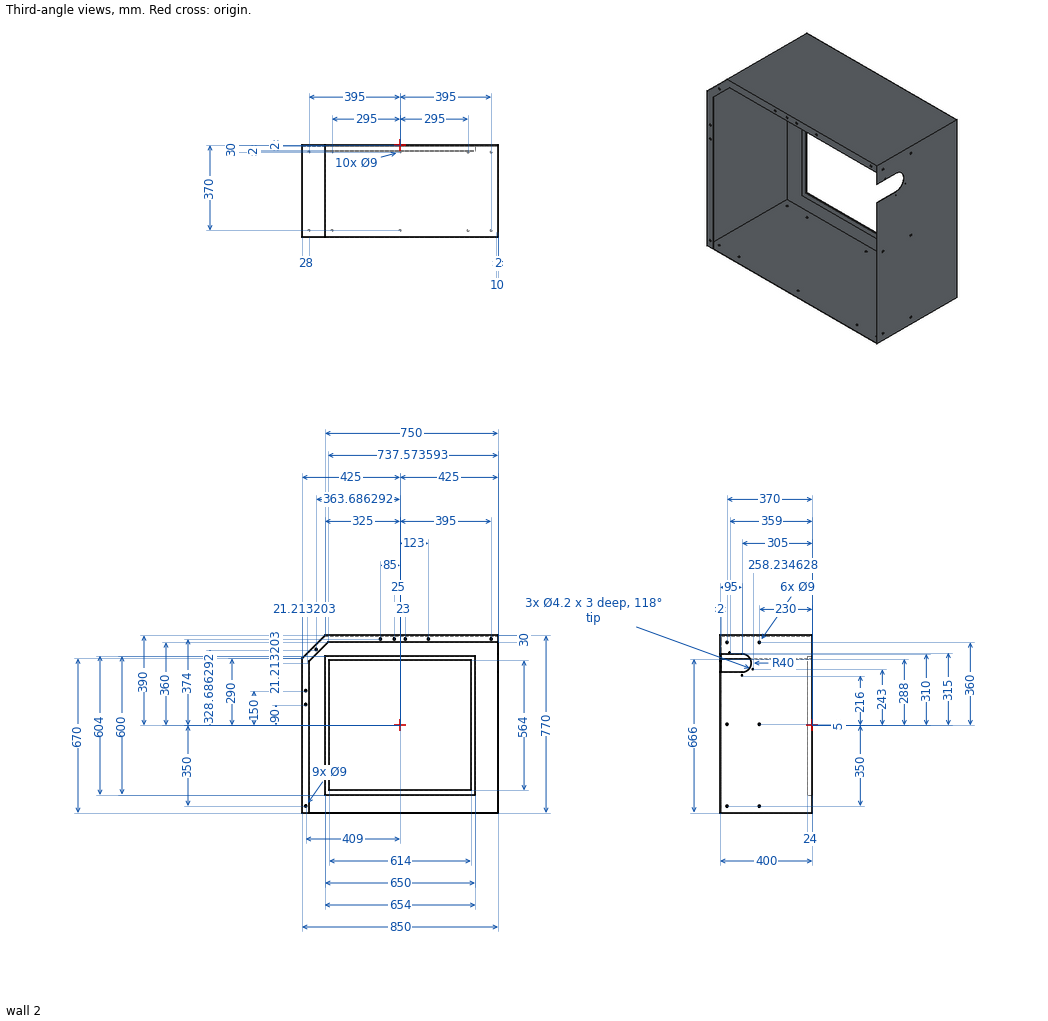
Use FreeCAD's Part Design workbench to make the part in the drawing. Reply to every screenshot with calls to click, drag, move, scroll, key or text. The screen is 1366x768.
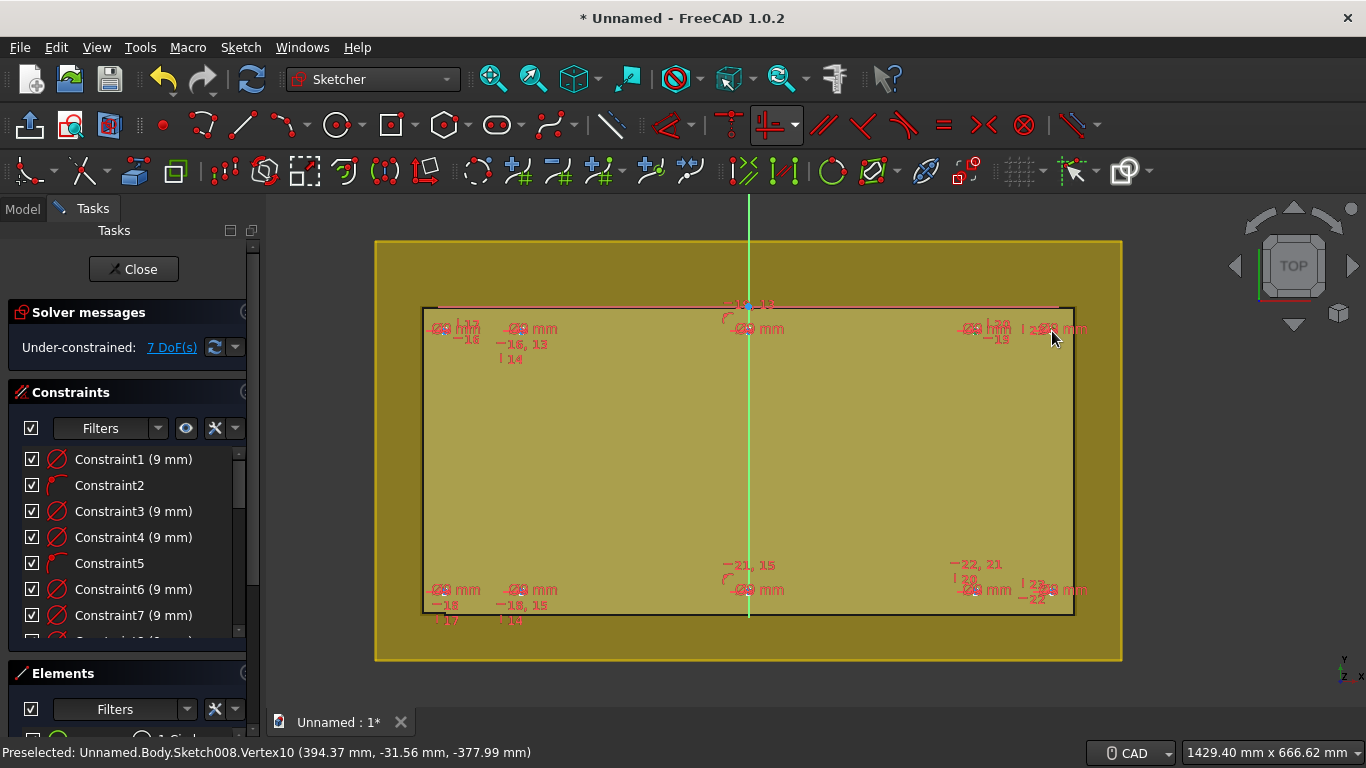
click(798, 126)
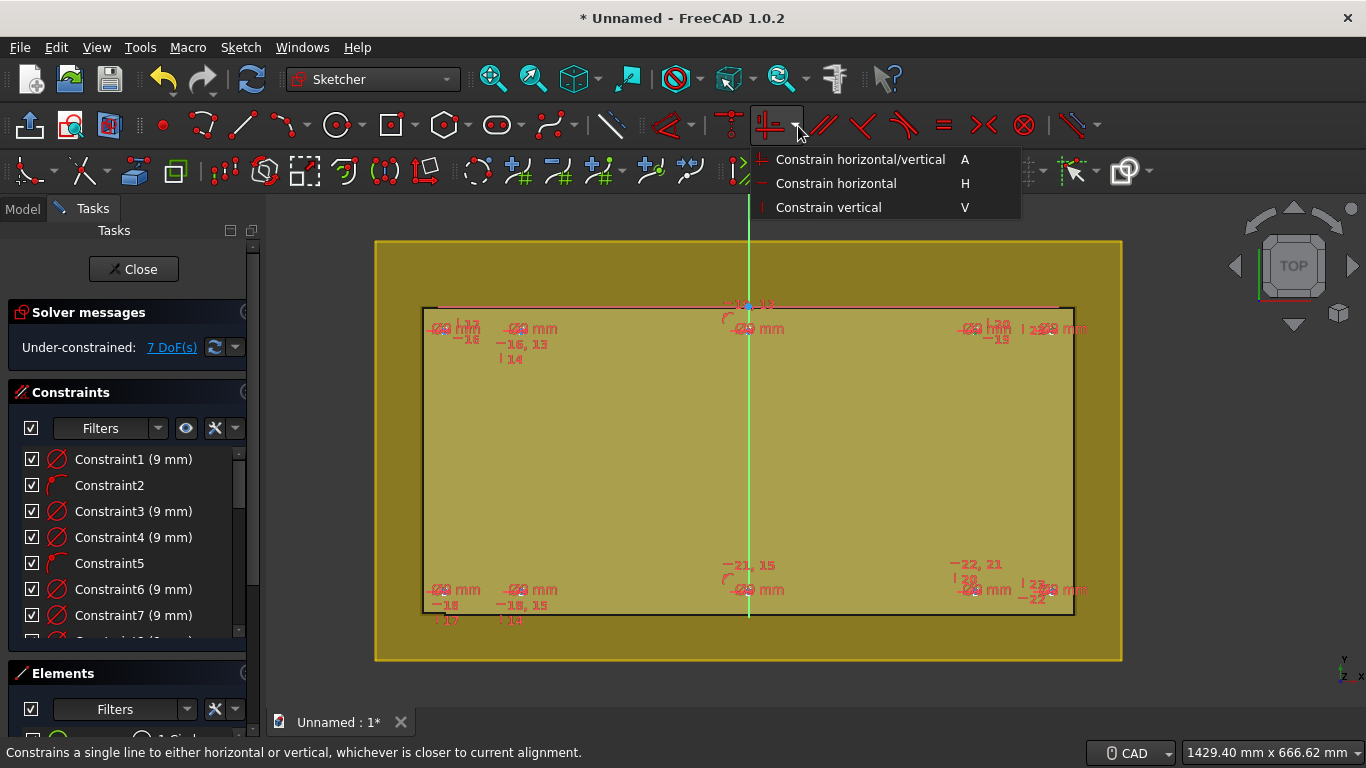
click(886, 183)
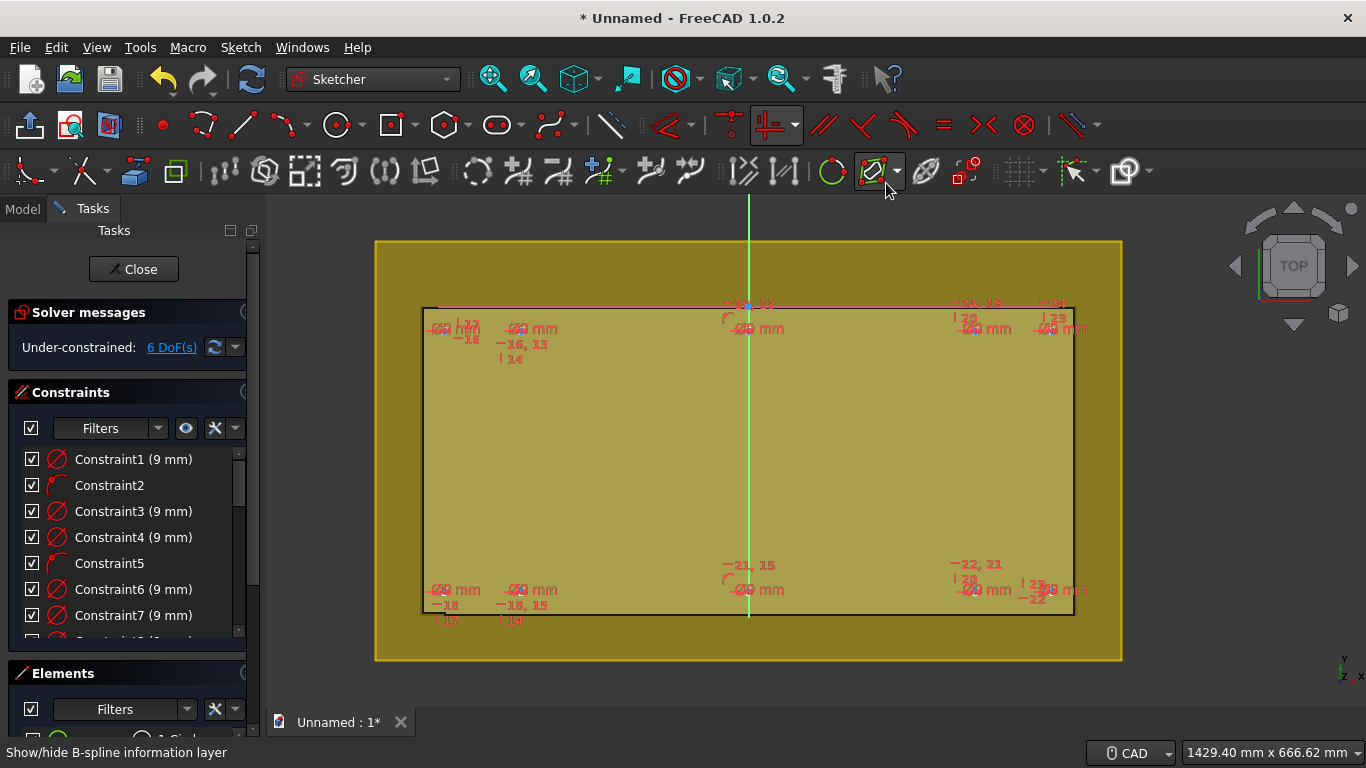
click(666, 126)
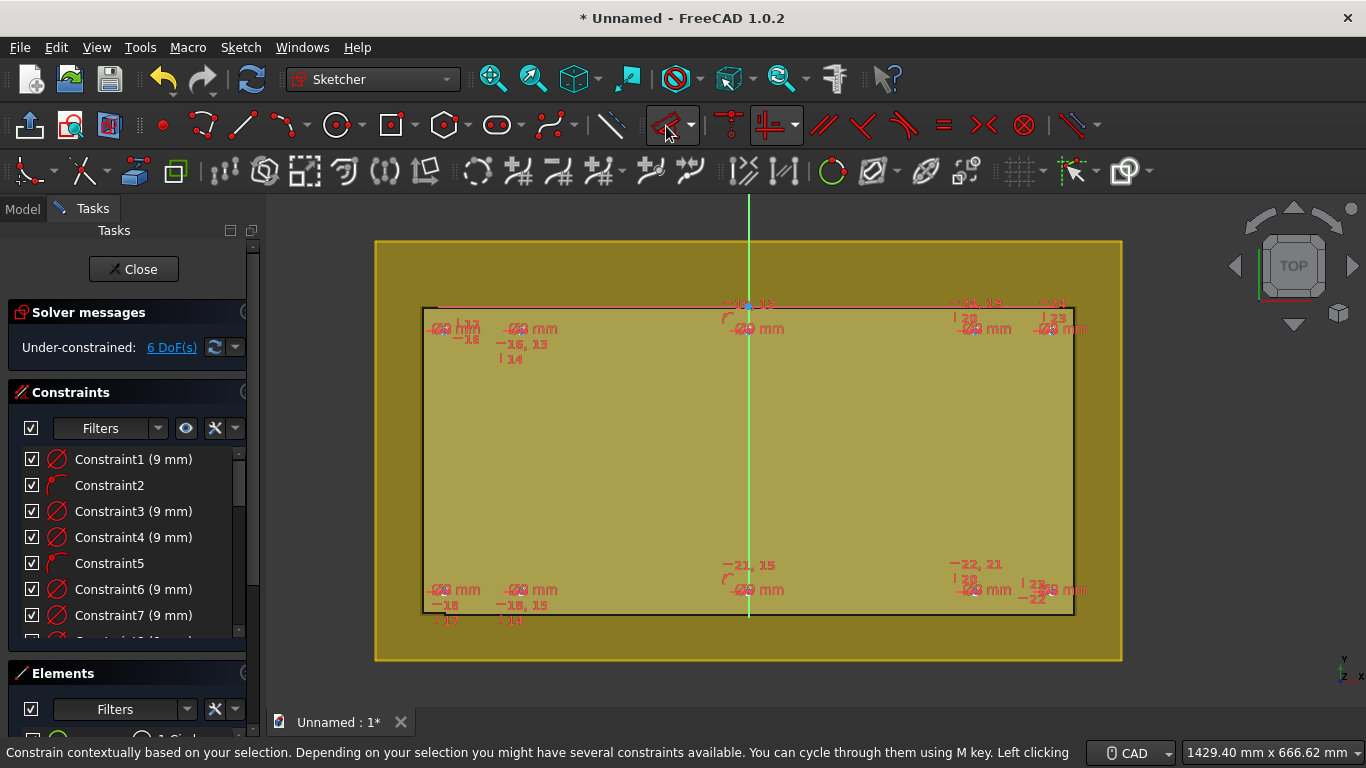
scroll(749, 331, up, 3)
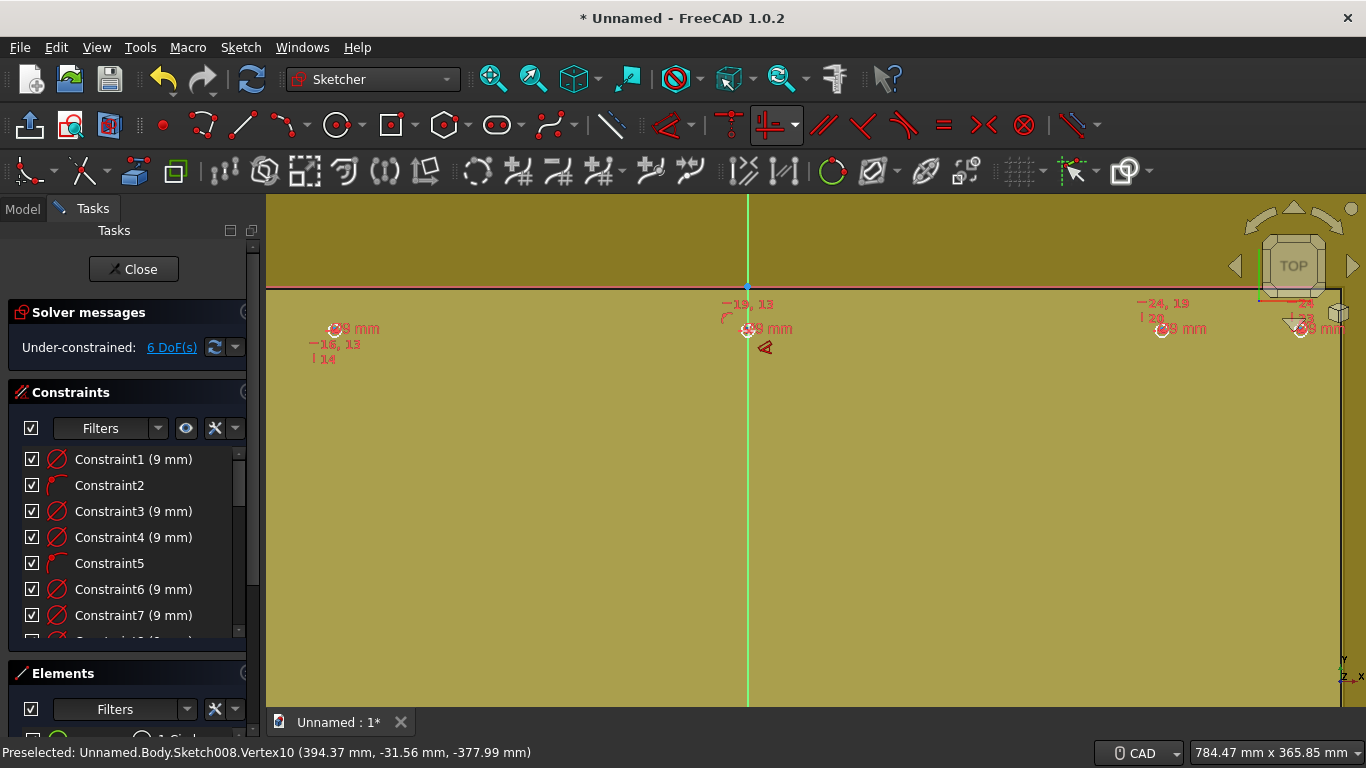
click(748, 331)
click(782, 309)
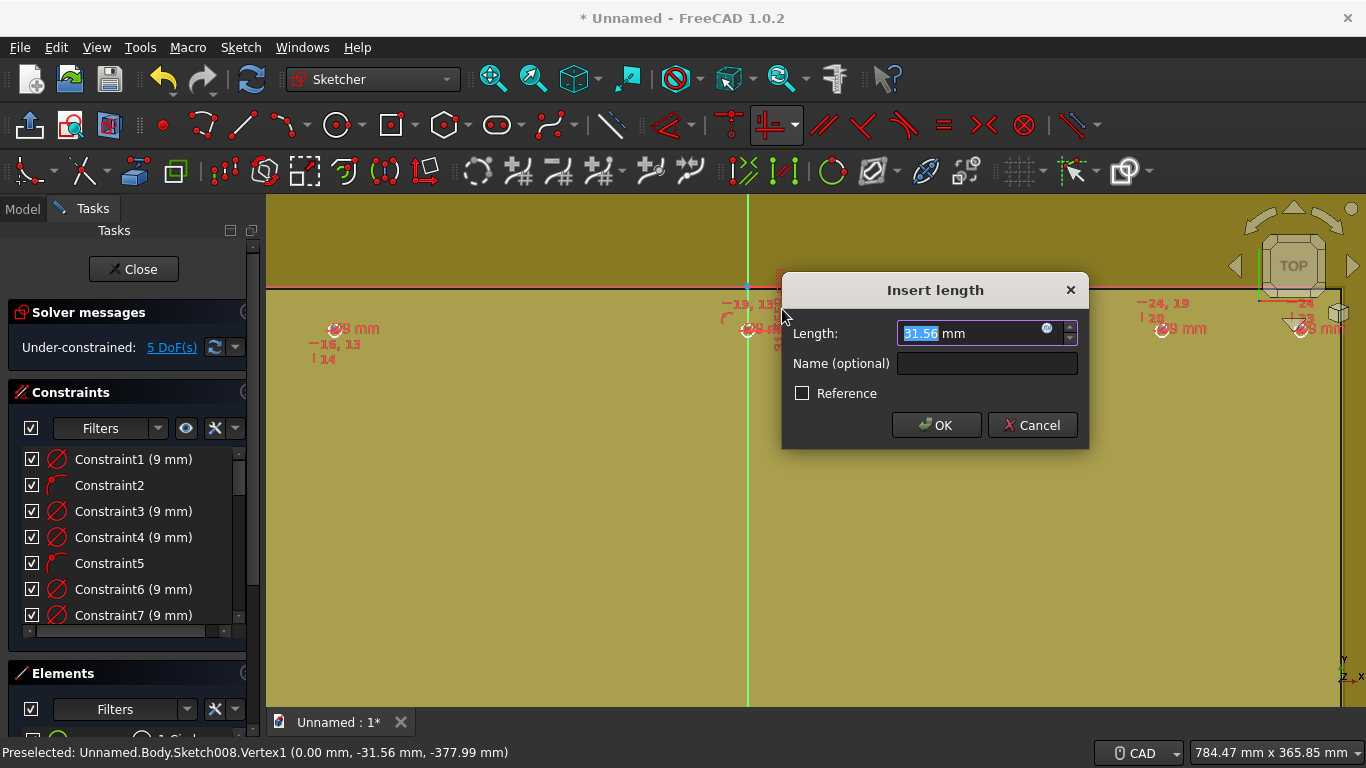
text(30)
key(Return)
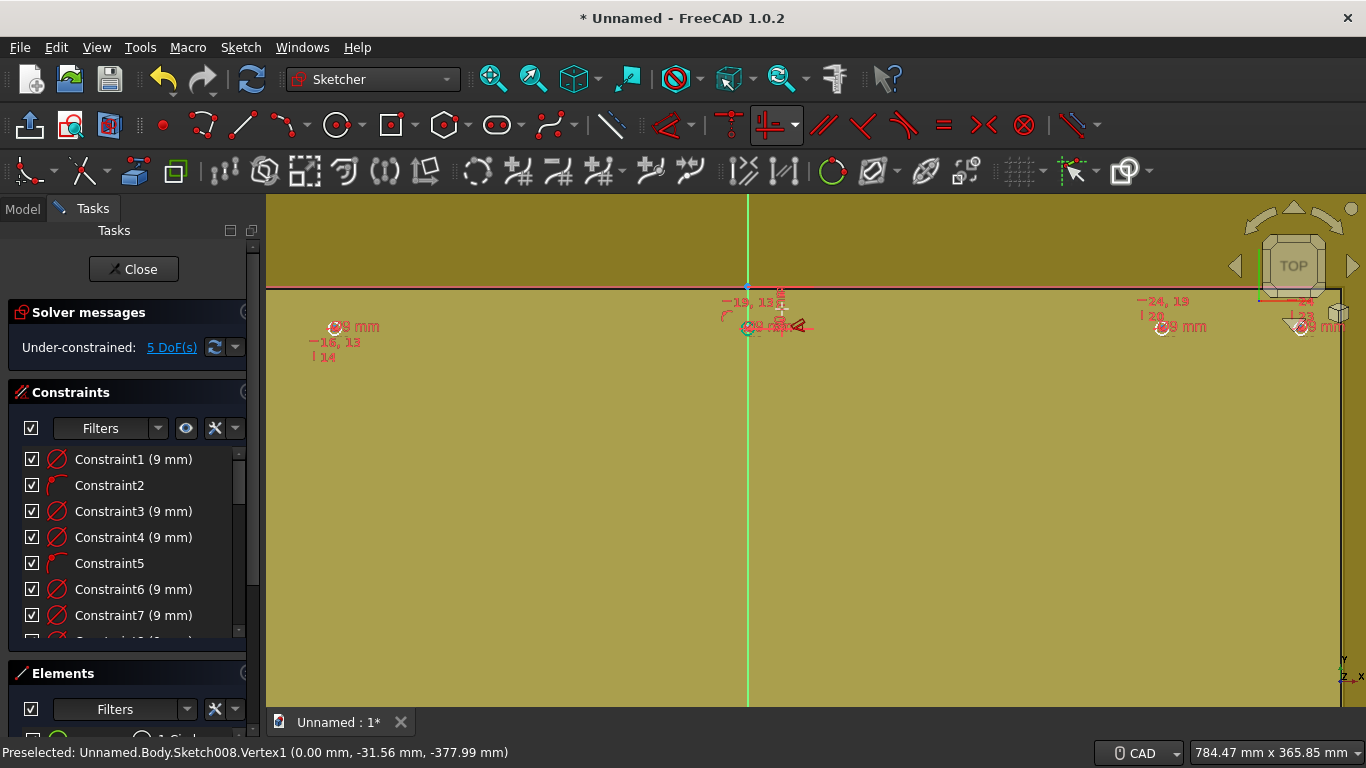
click(335, 329)
click(541, 253)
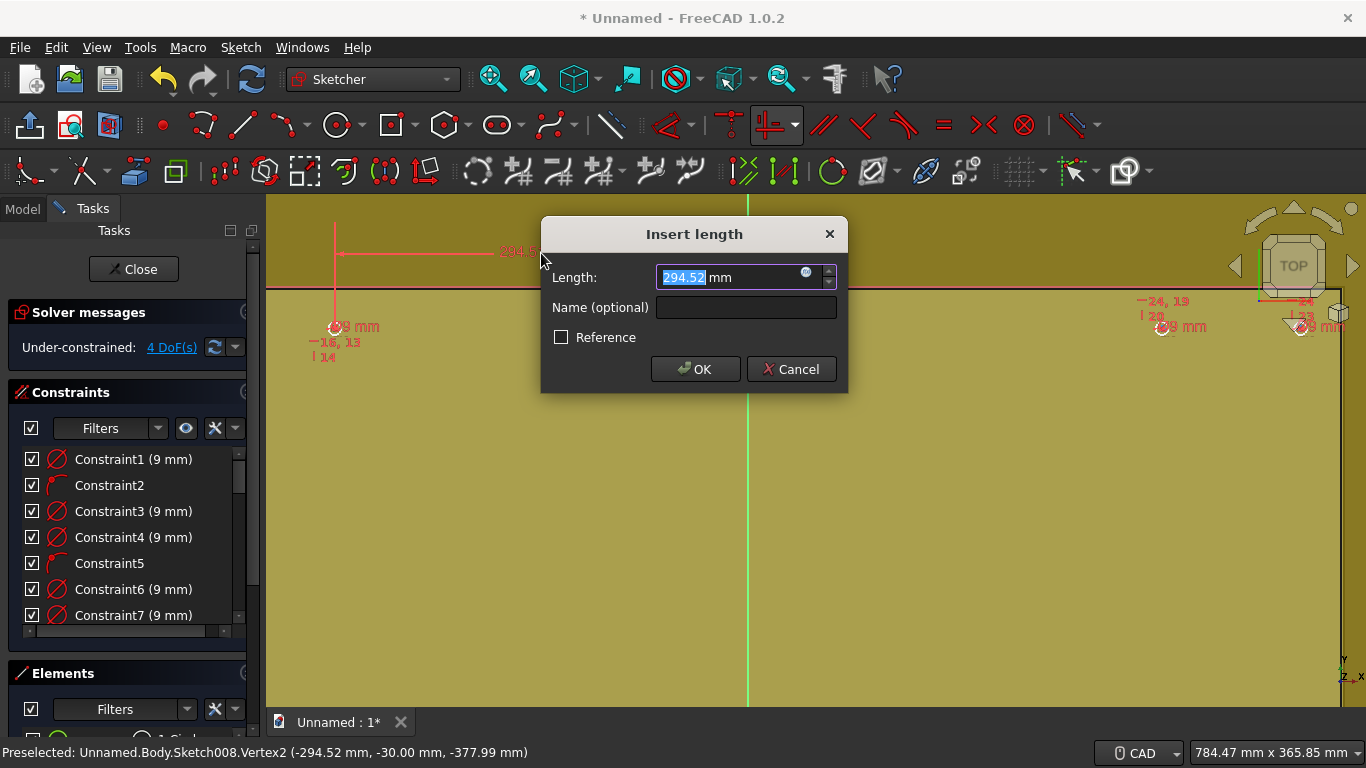
text(295)
key(Return)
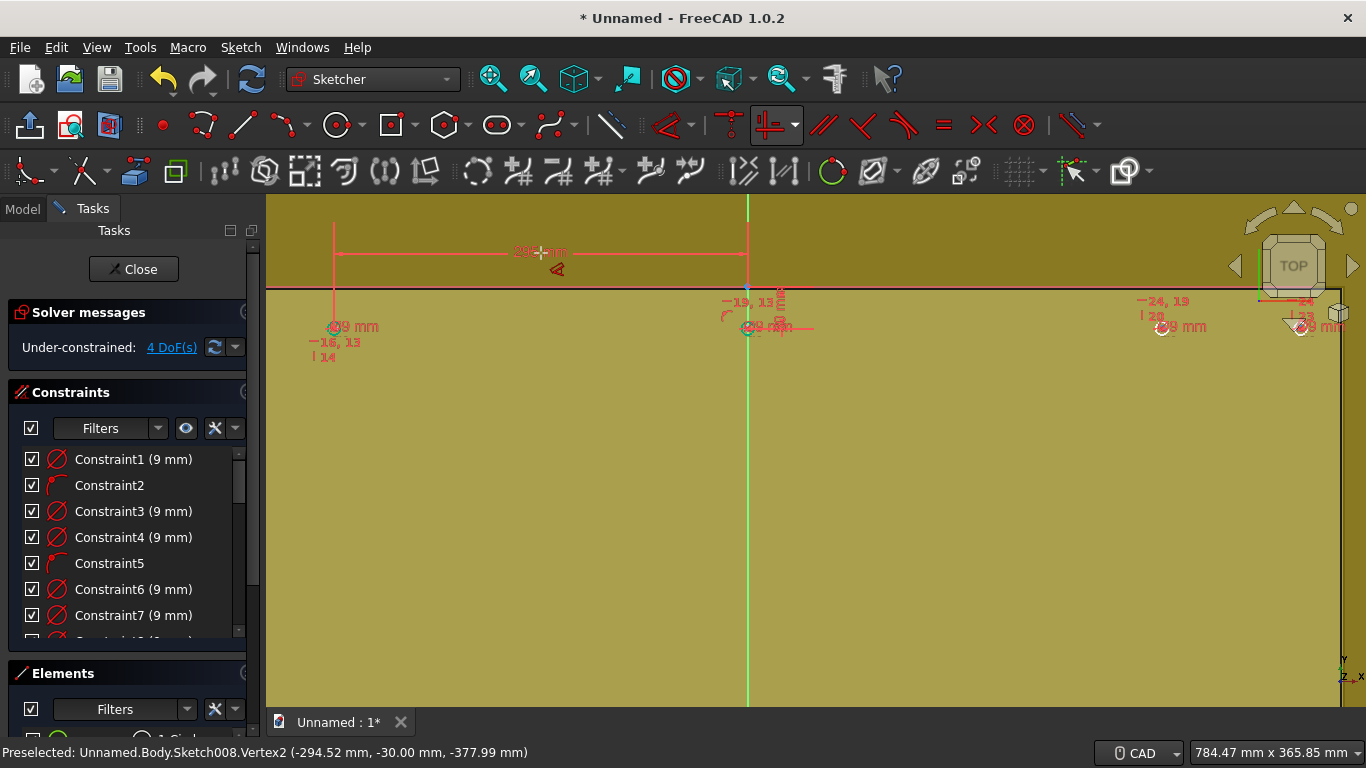
scroll(747, 331, down, 3)